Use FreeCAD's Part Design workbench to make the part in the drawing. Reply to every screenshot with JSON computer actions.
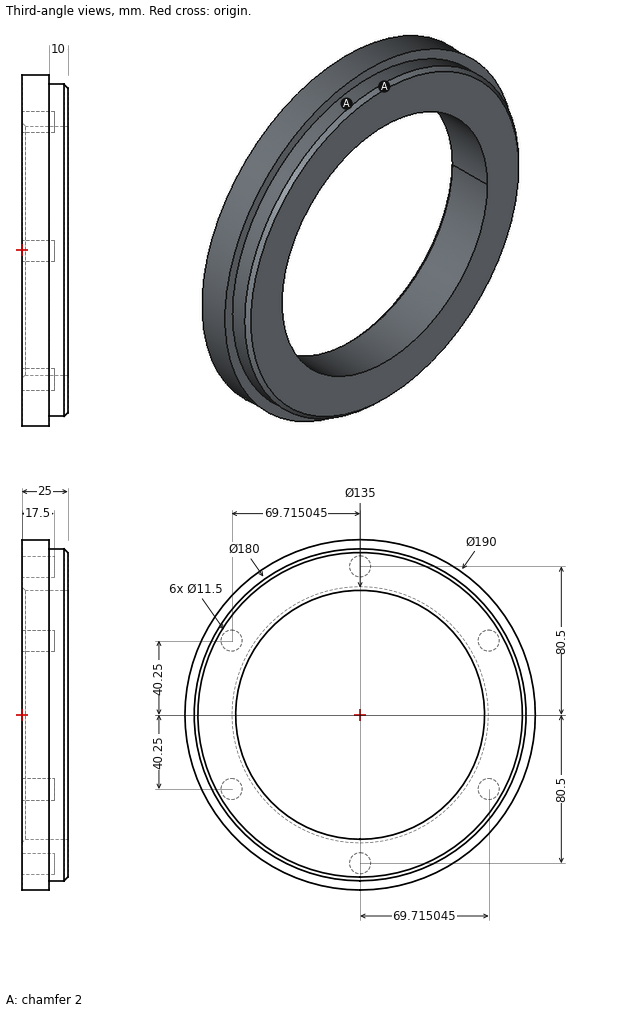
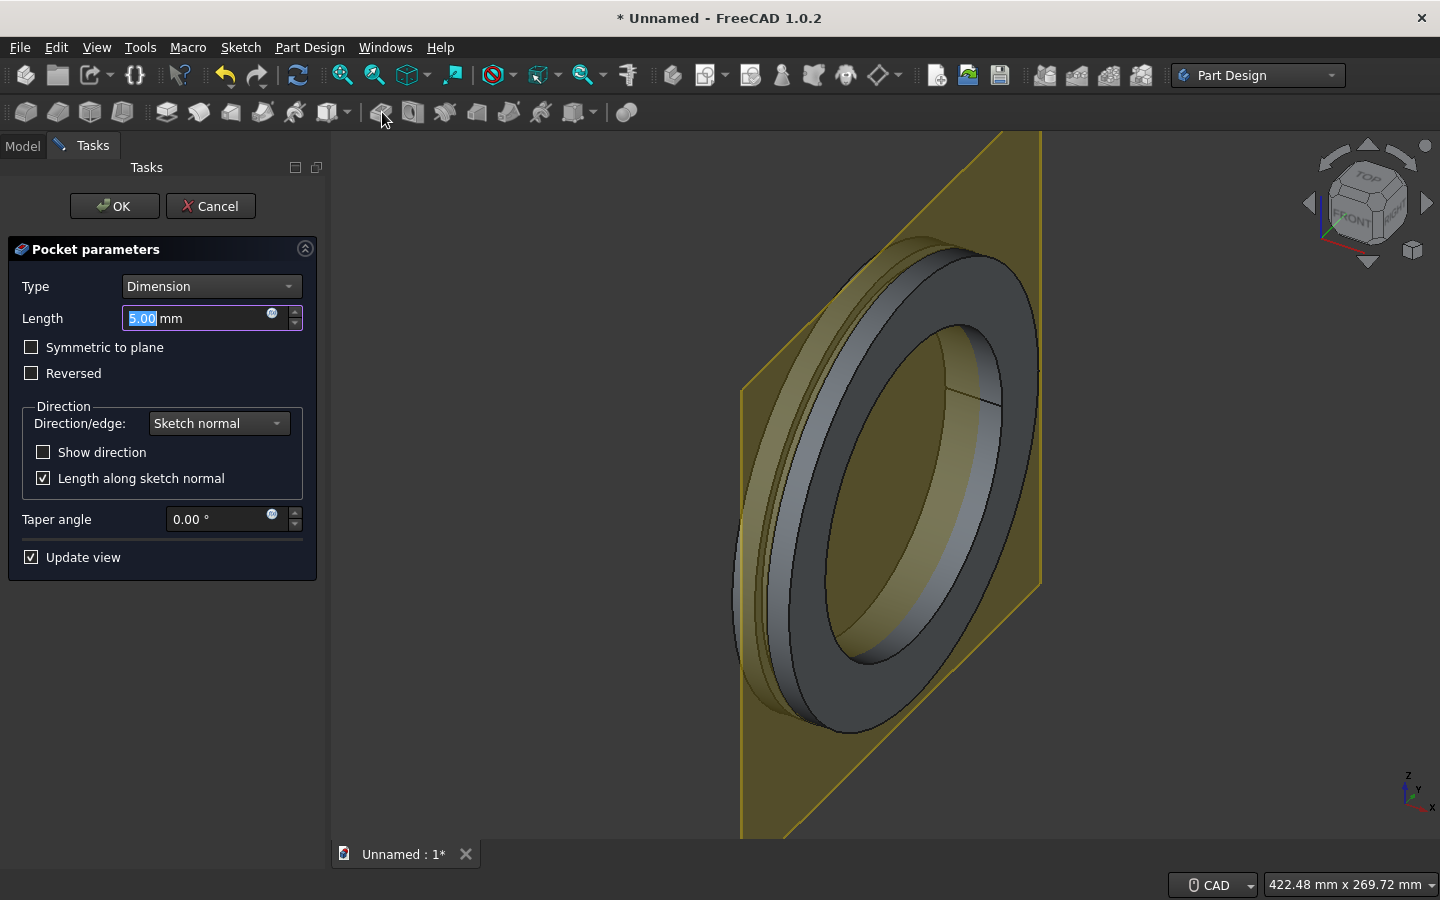
{"action": "type", "text": "10"}
{"action": "key", "text": "Tab"}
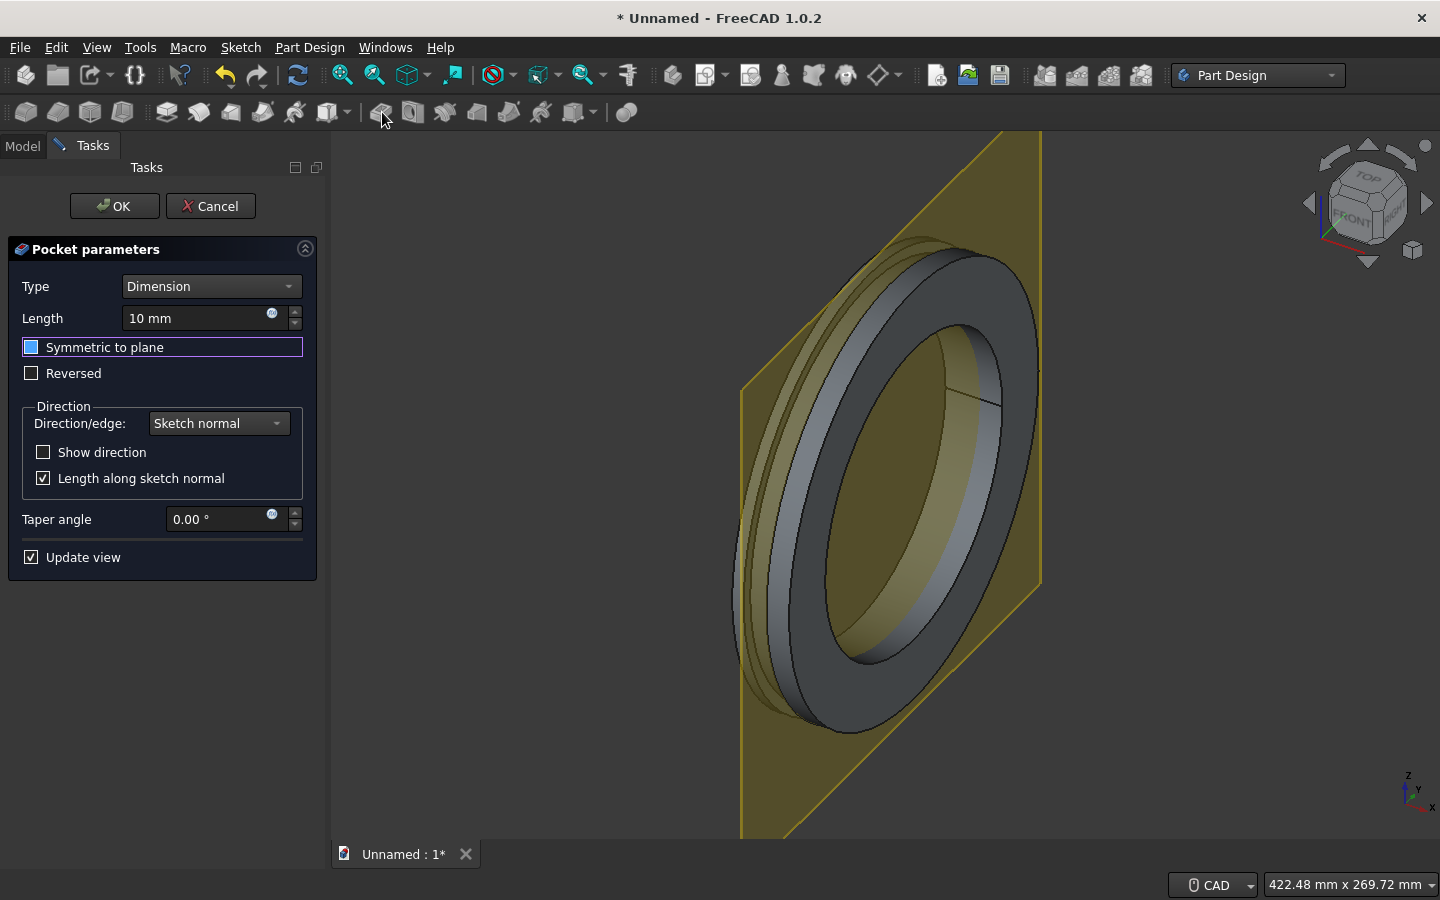
{"action": "left_click", "coordinate": [30, 373]}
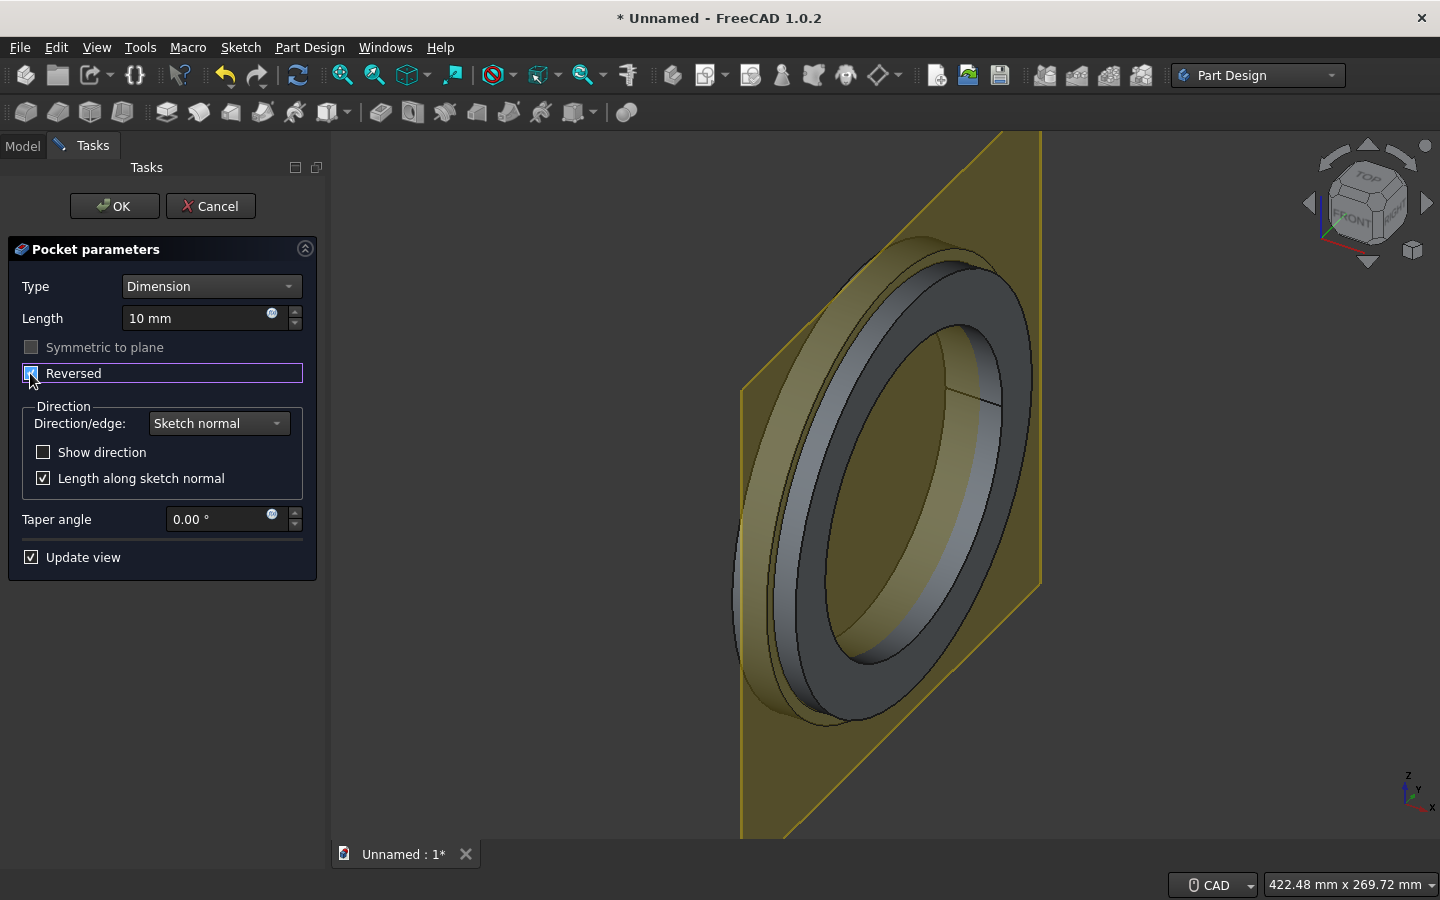
{"action": "left_click", "coordinate": [115, 206]}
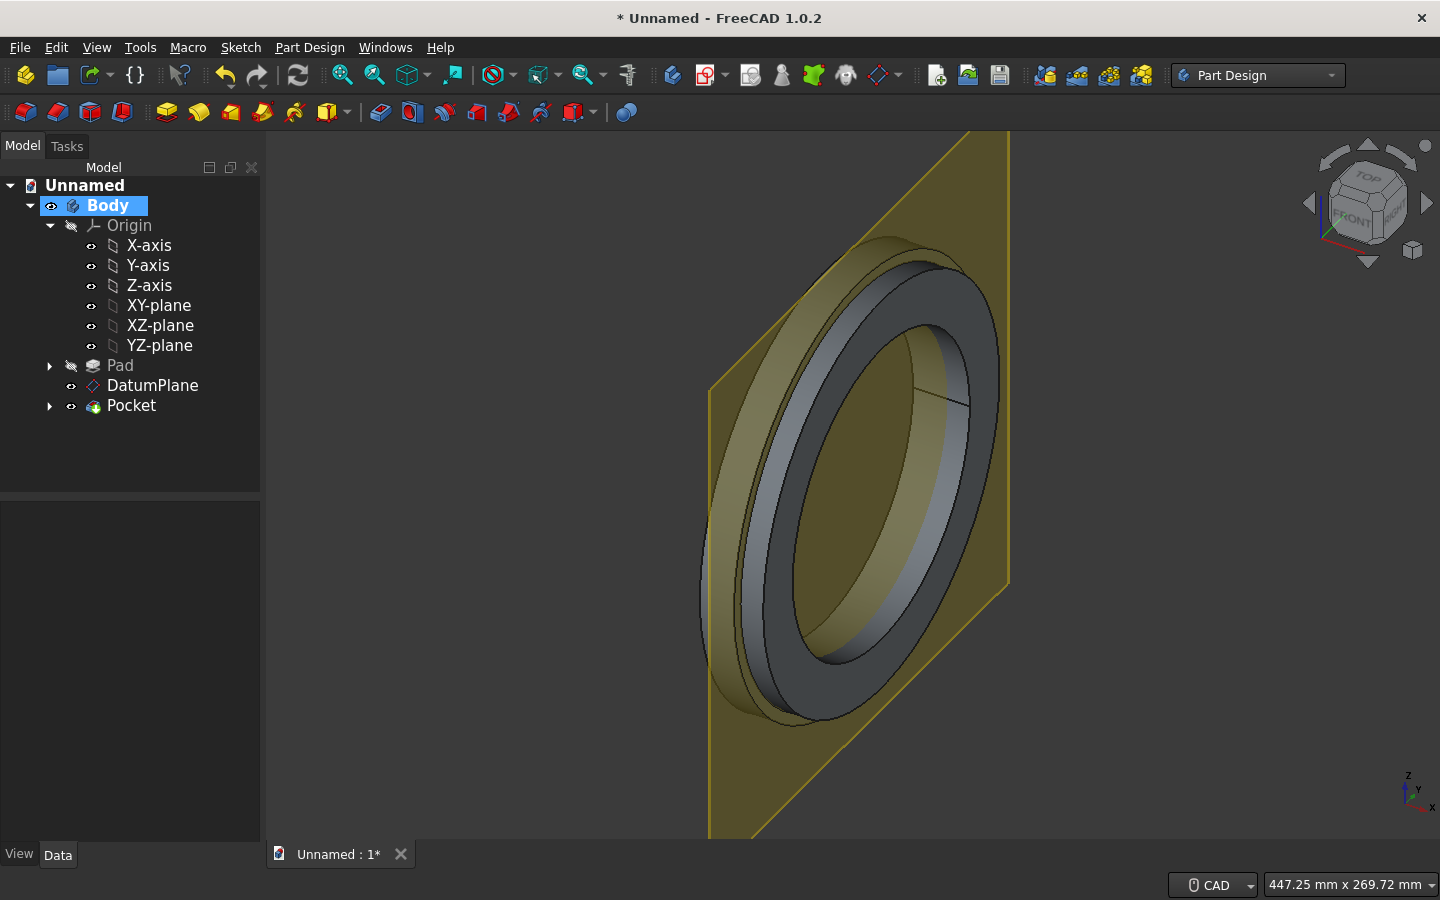
{"action": "left_click", "coordinate": [116, 386]}
{"action": "key", "text": "space"}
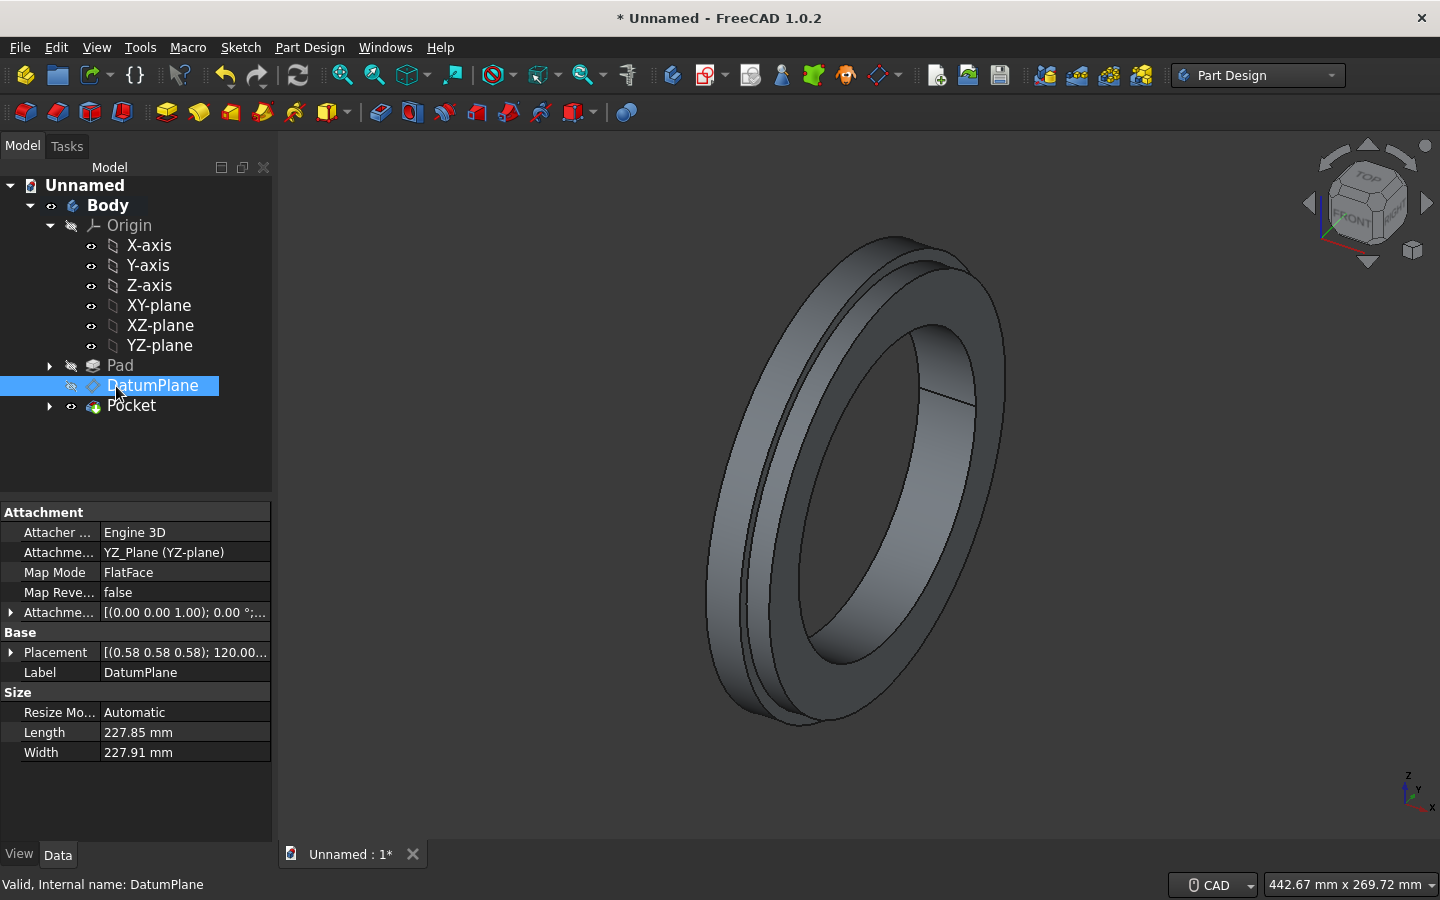
{"action": "left_click", "coordinate": [318, 799]}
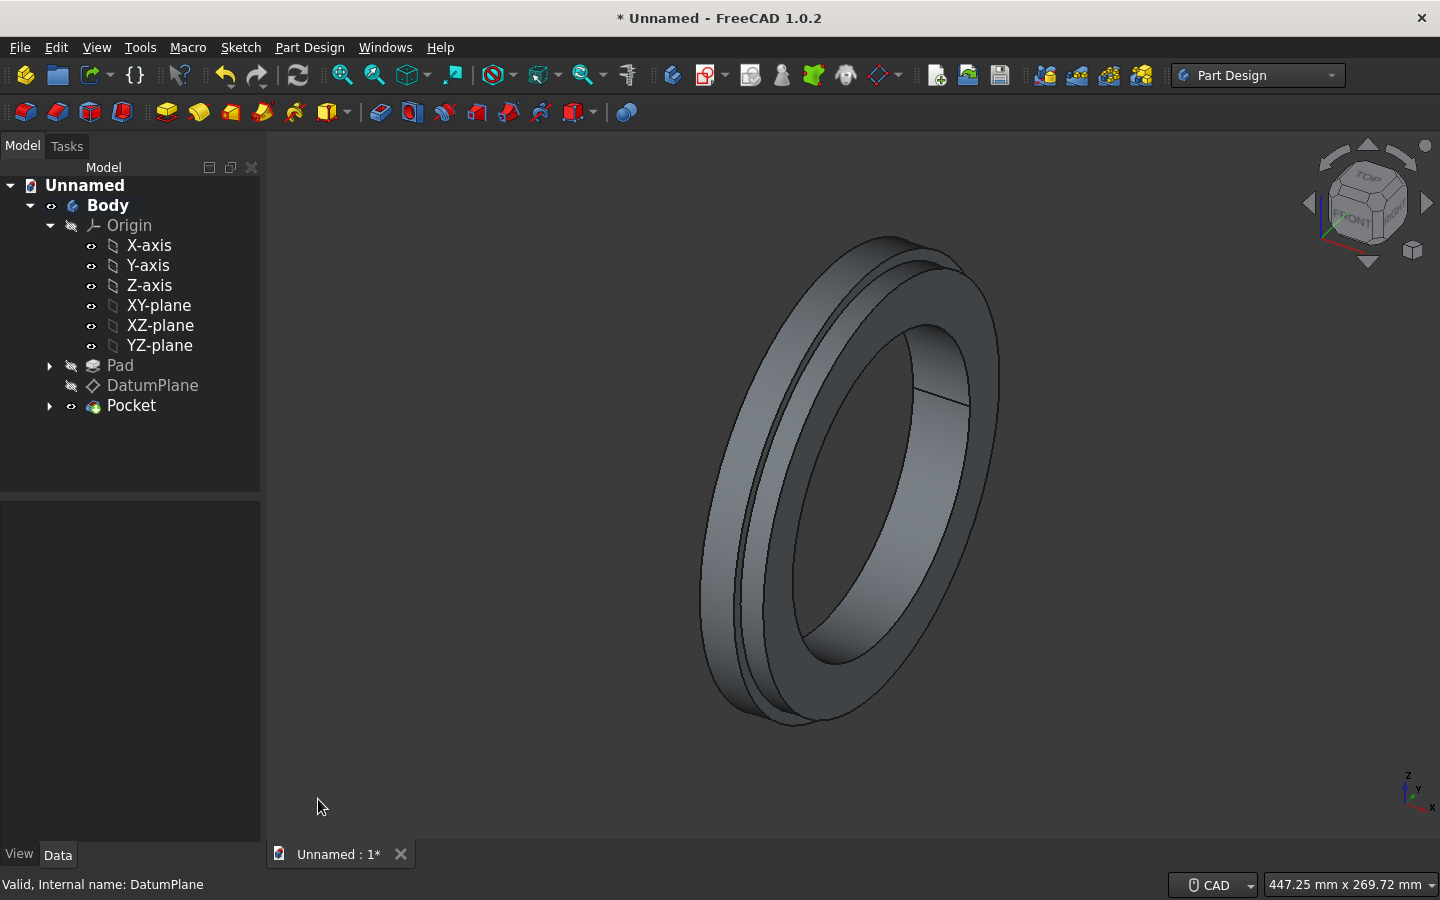
{"action": "left_click", "coordinate": [706, 76]}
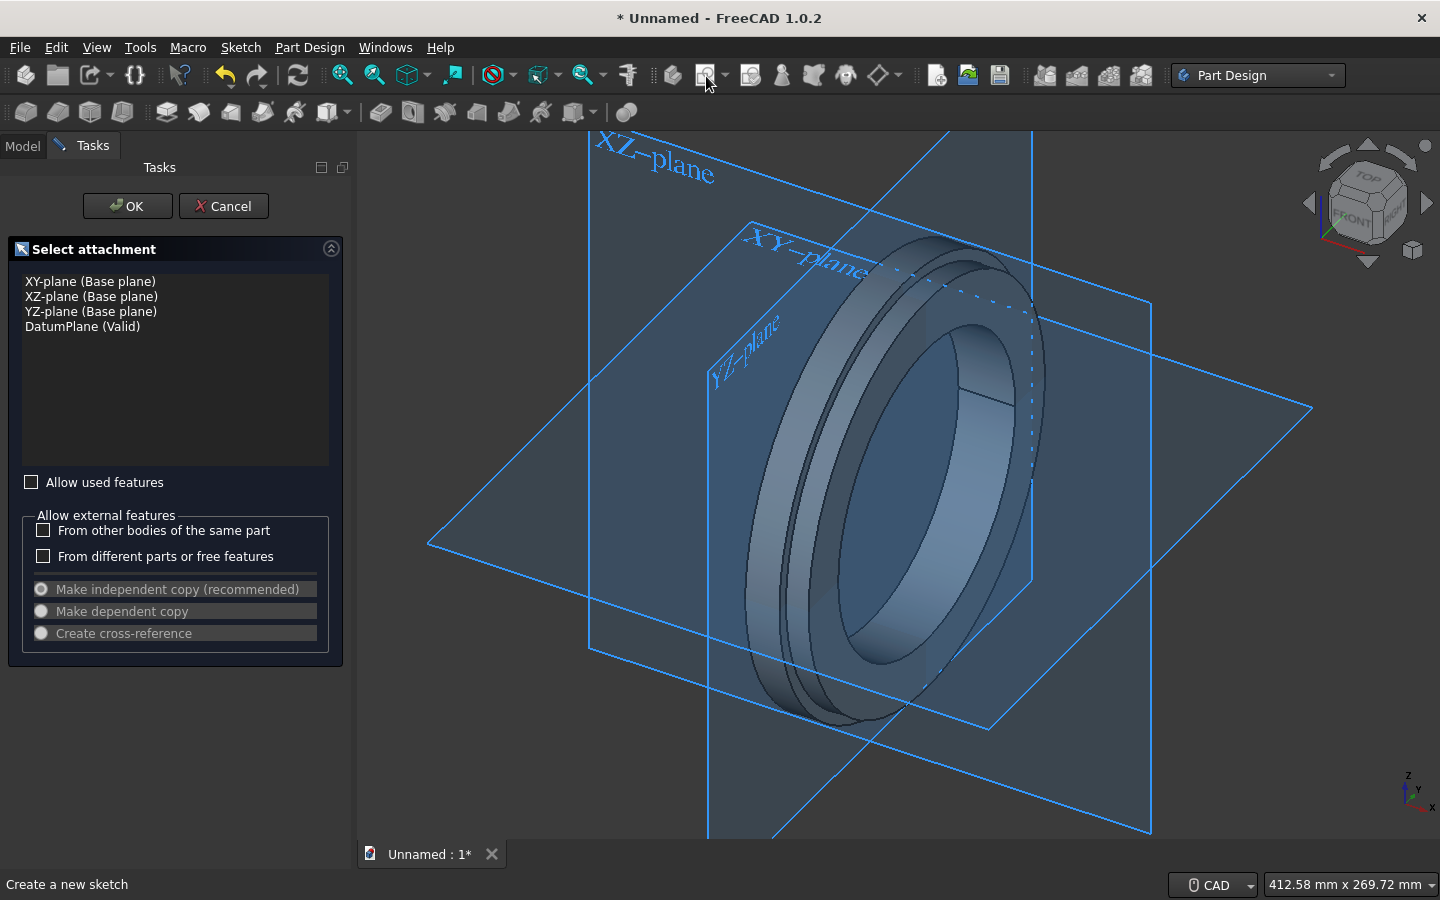
{"action": "left_click", "coordinate": [82, 312]}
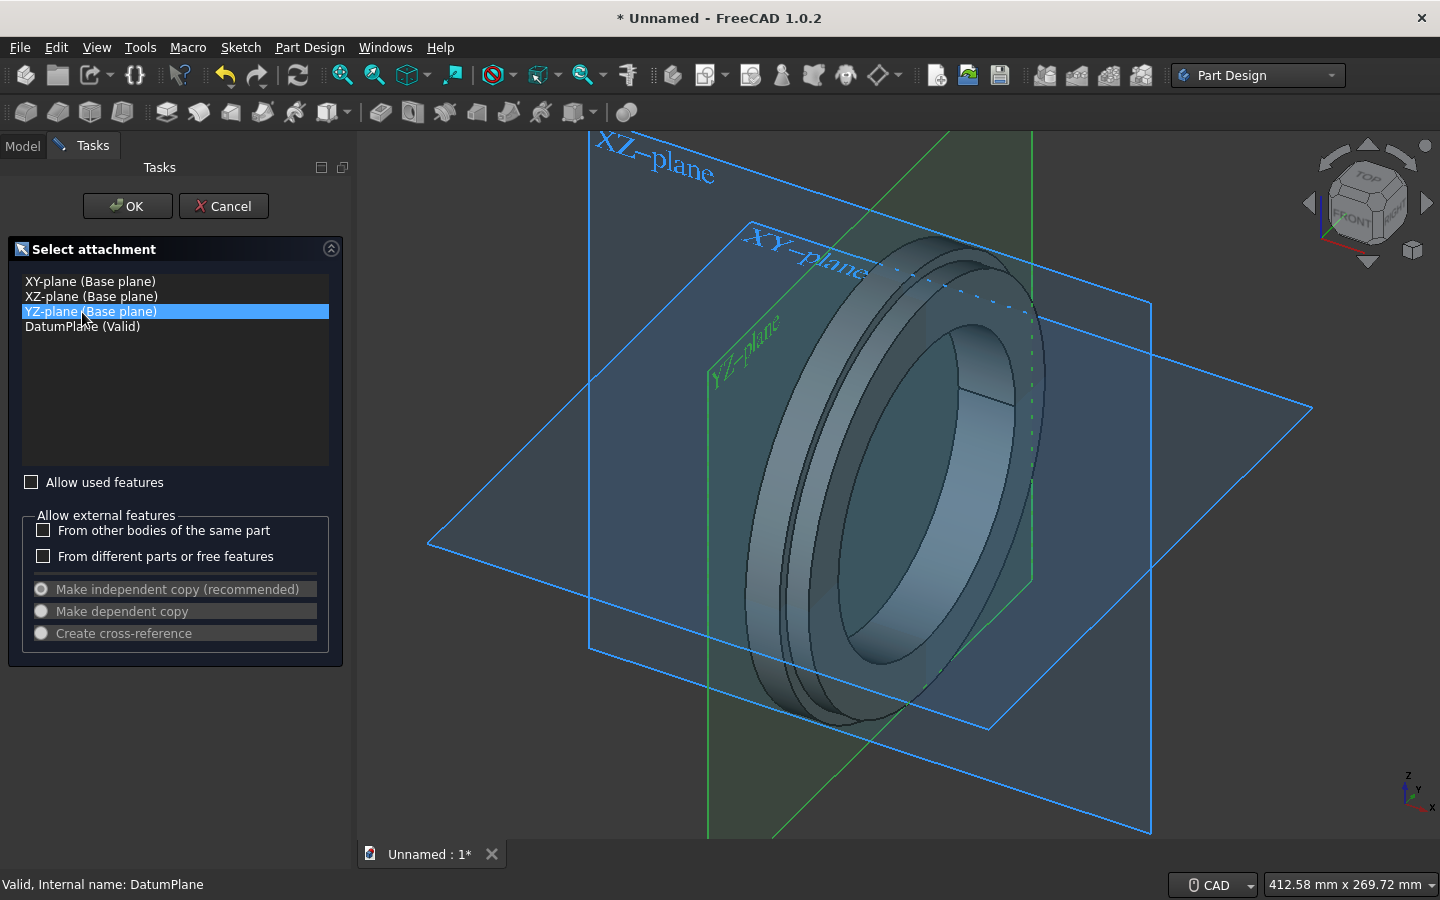
{"action": "left_click", "coordinate": [128, 206]}